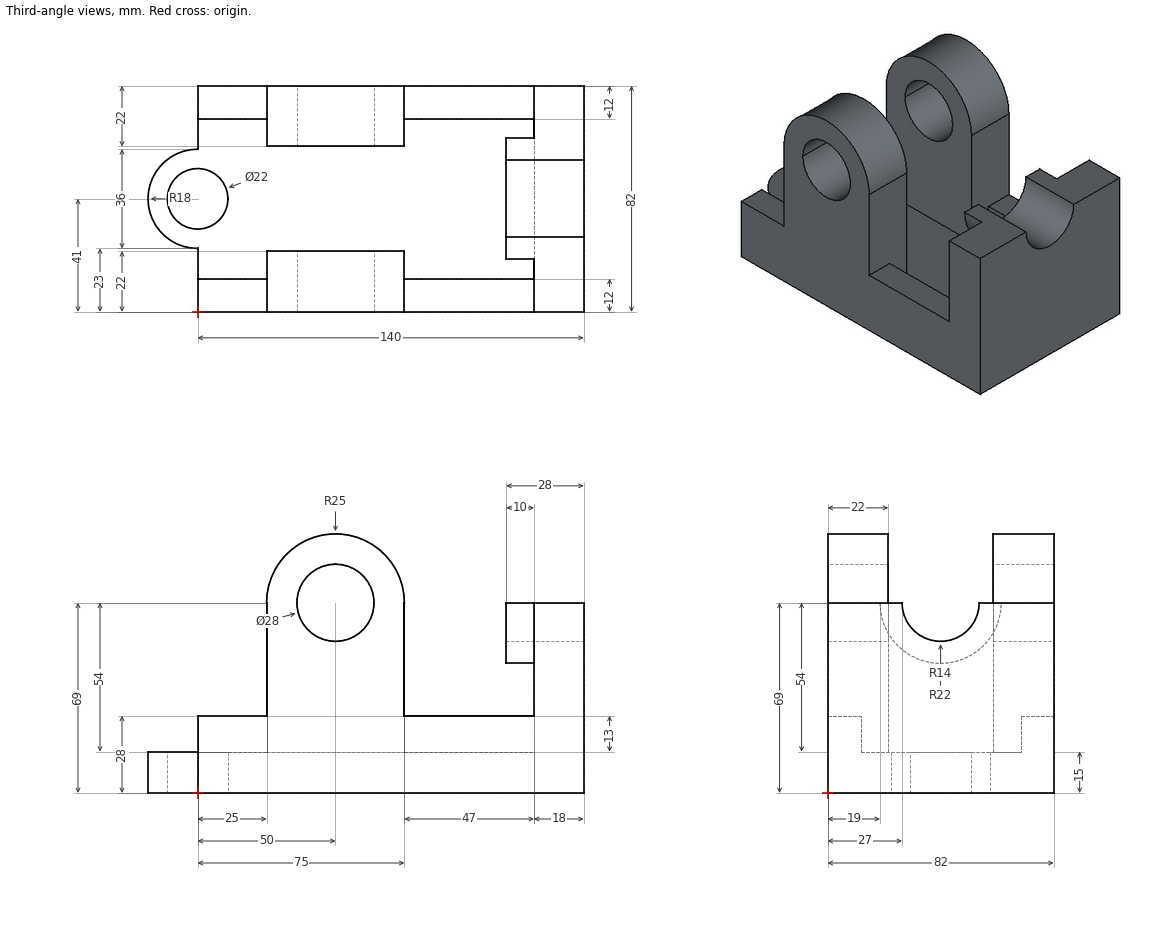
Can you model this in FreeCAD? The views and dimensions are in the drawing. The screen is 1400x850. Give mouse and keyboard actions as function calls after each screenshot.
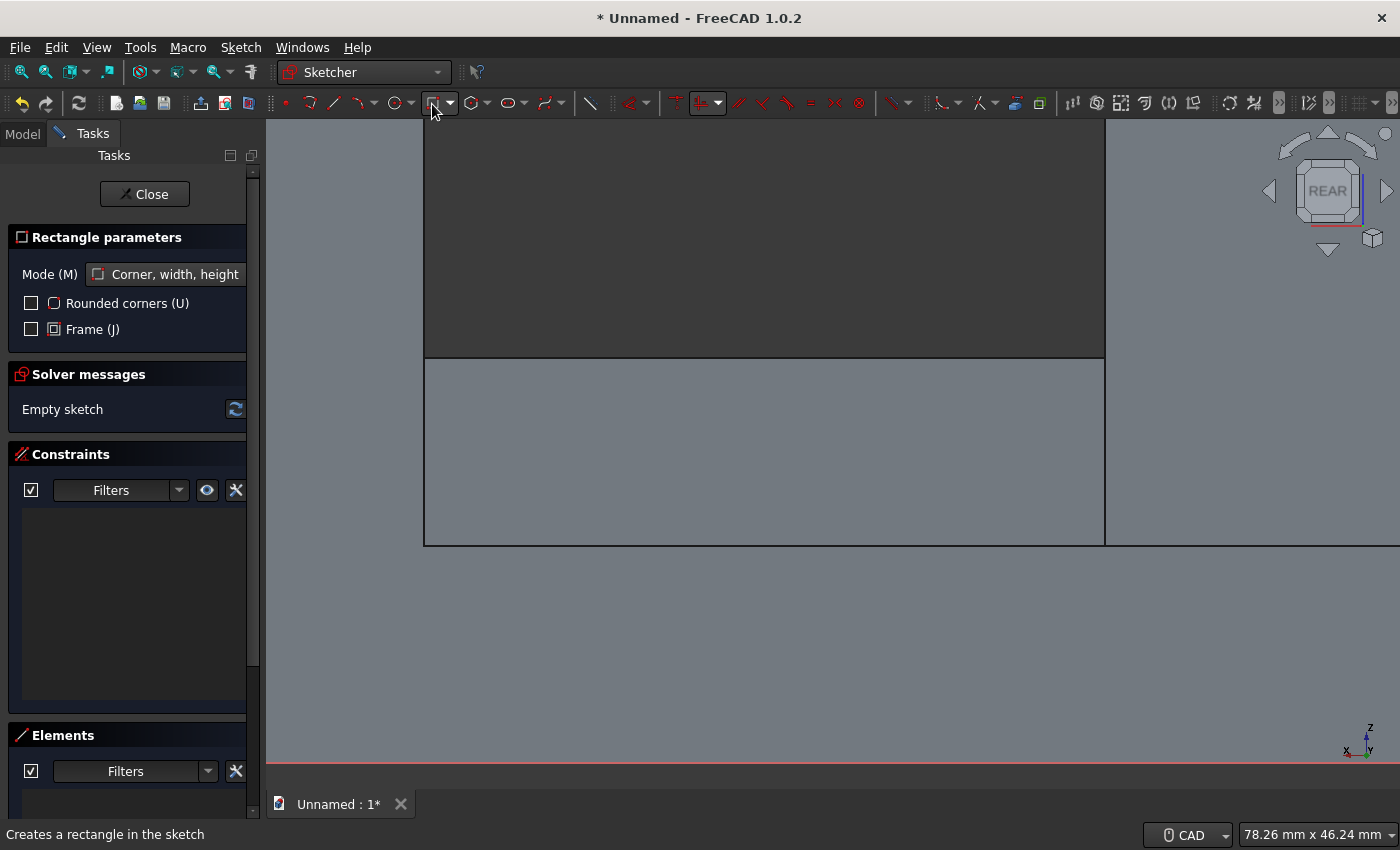
click(424, 358)
click(1105, 546)
key(Escape)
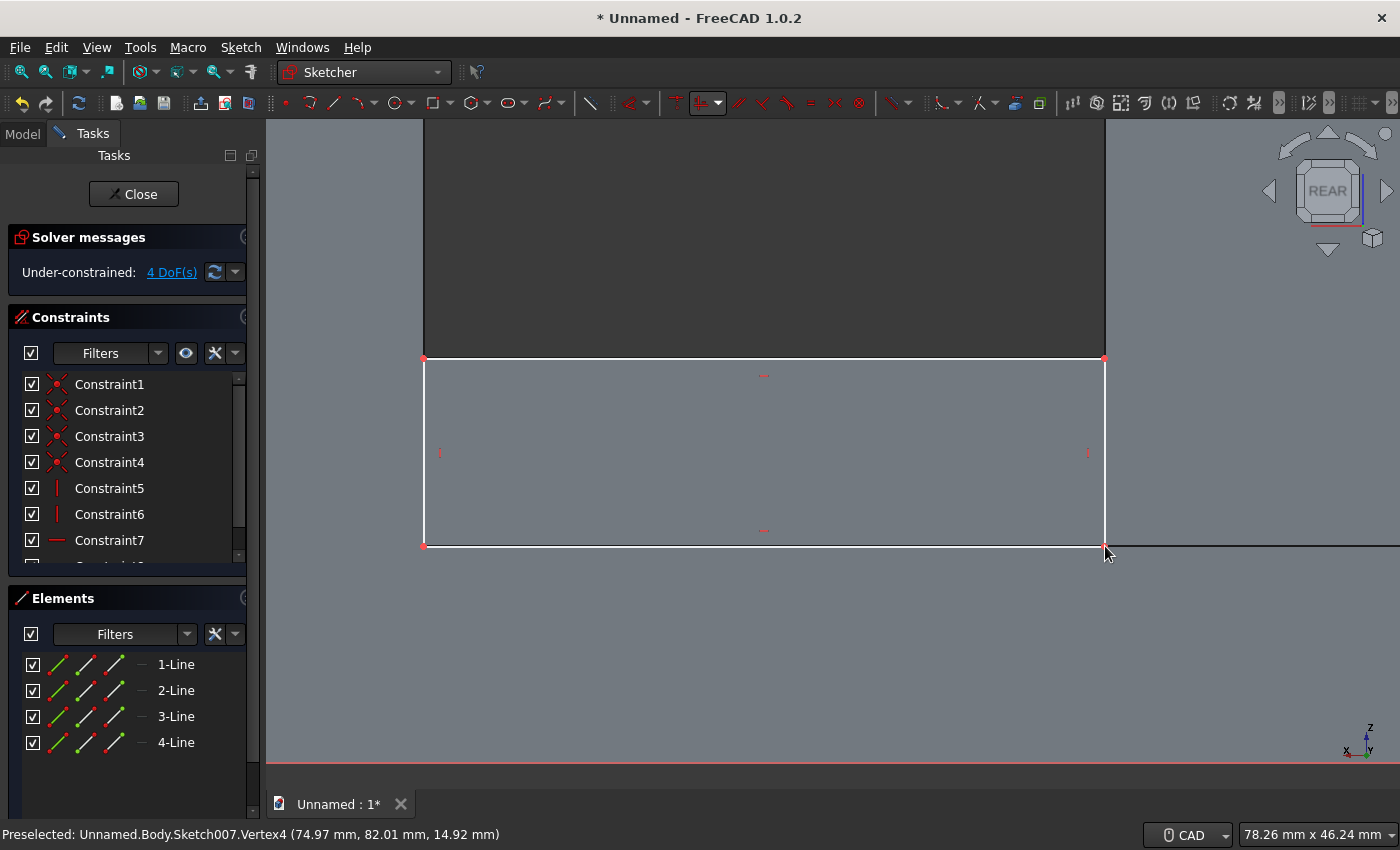
click(630, 104)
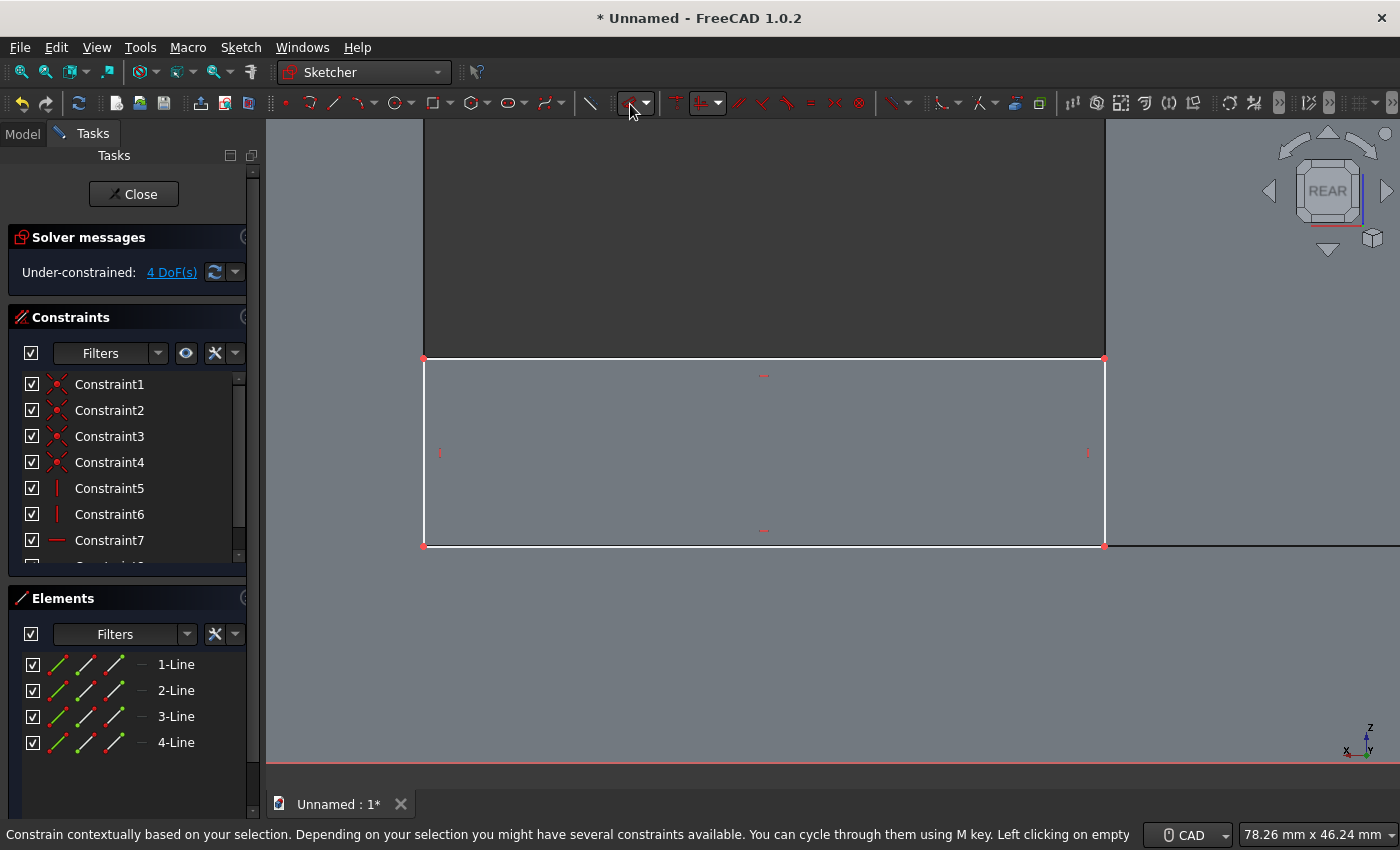
click(424, 415)
click(390, 453)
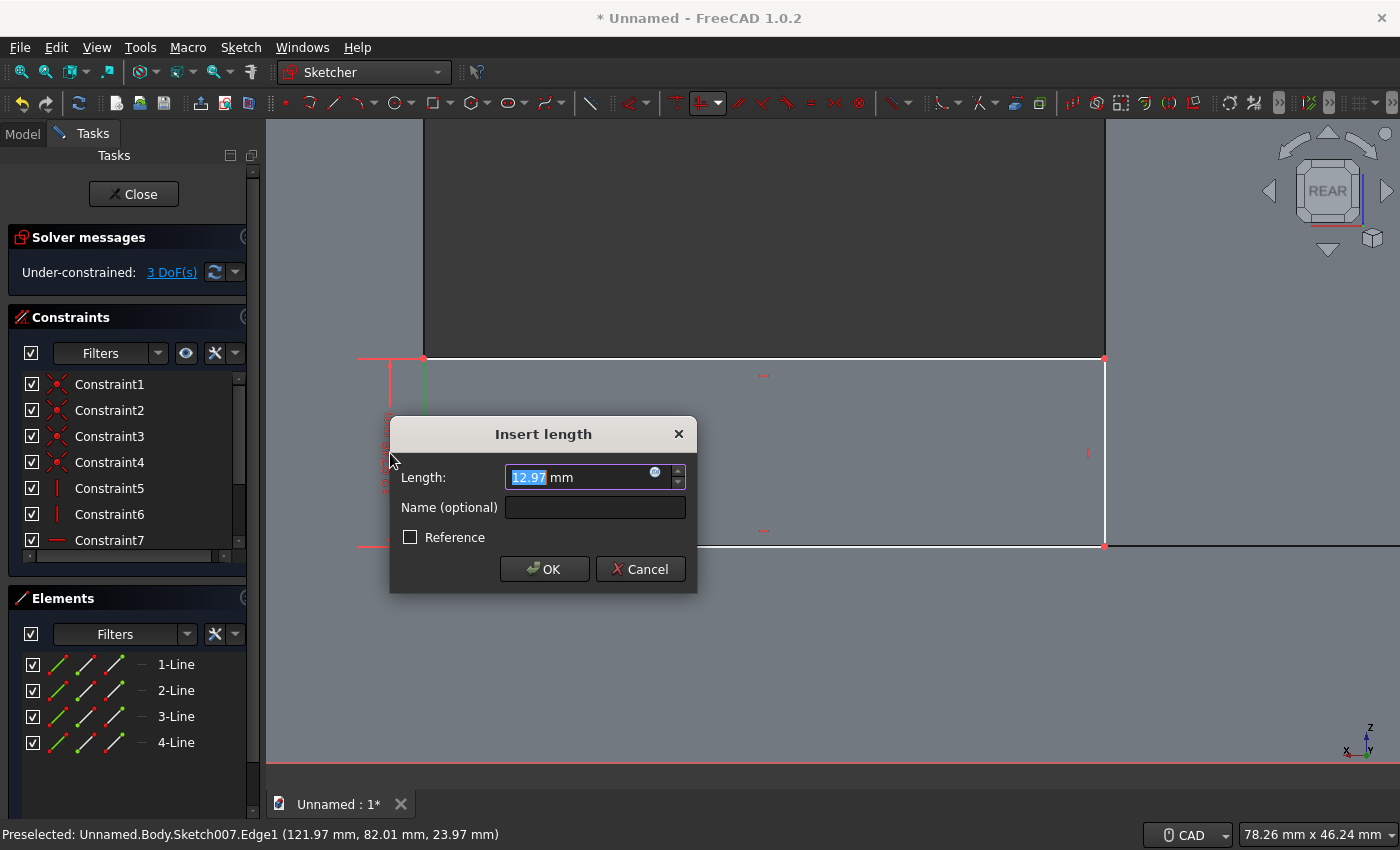
text(13)
key(Return)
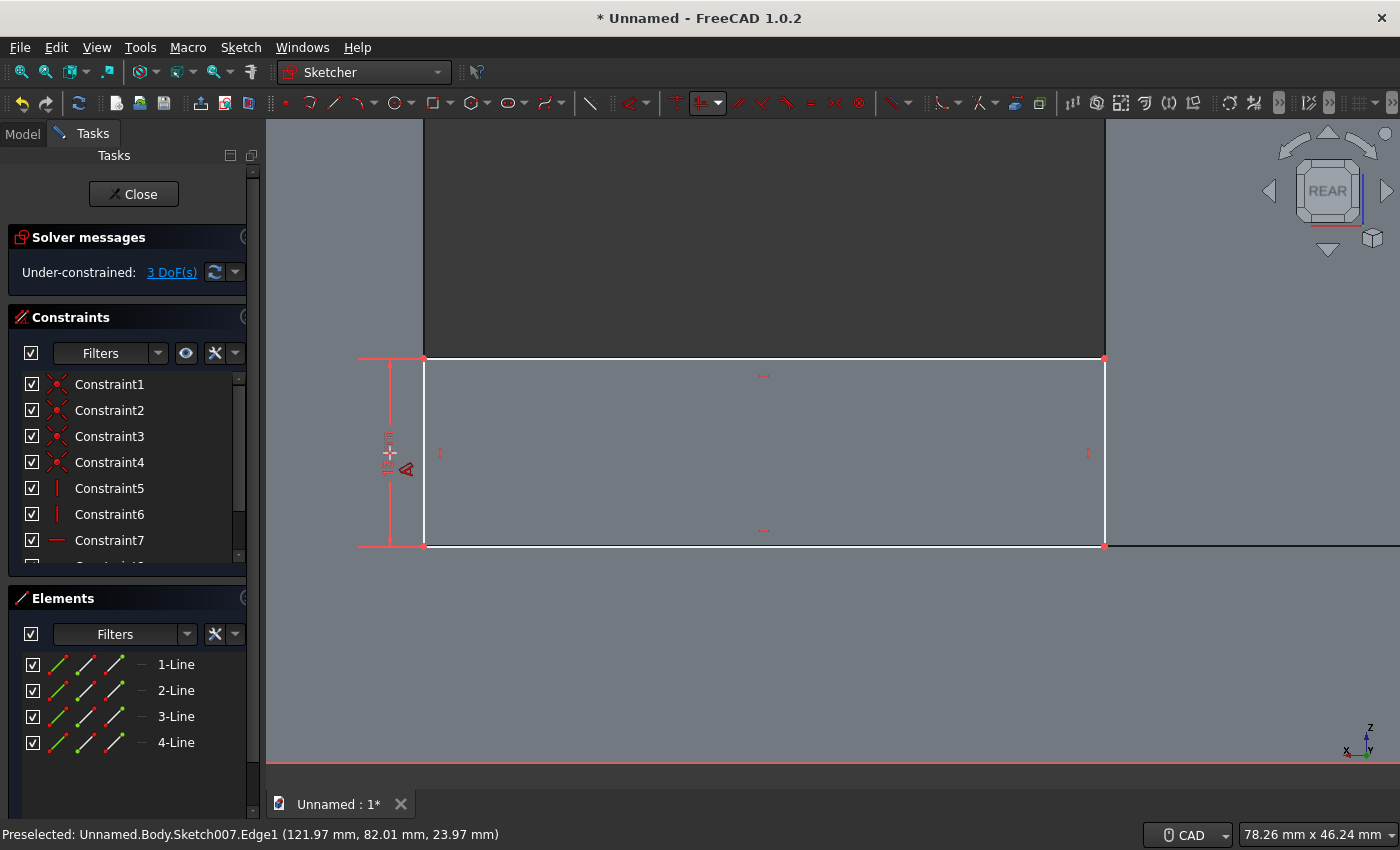
click(628, 547)
click(765, 581)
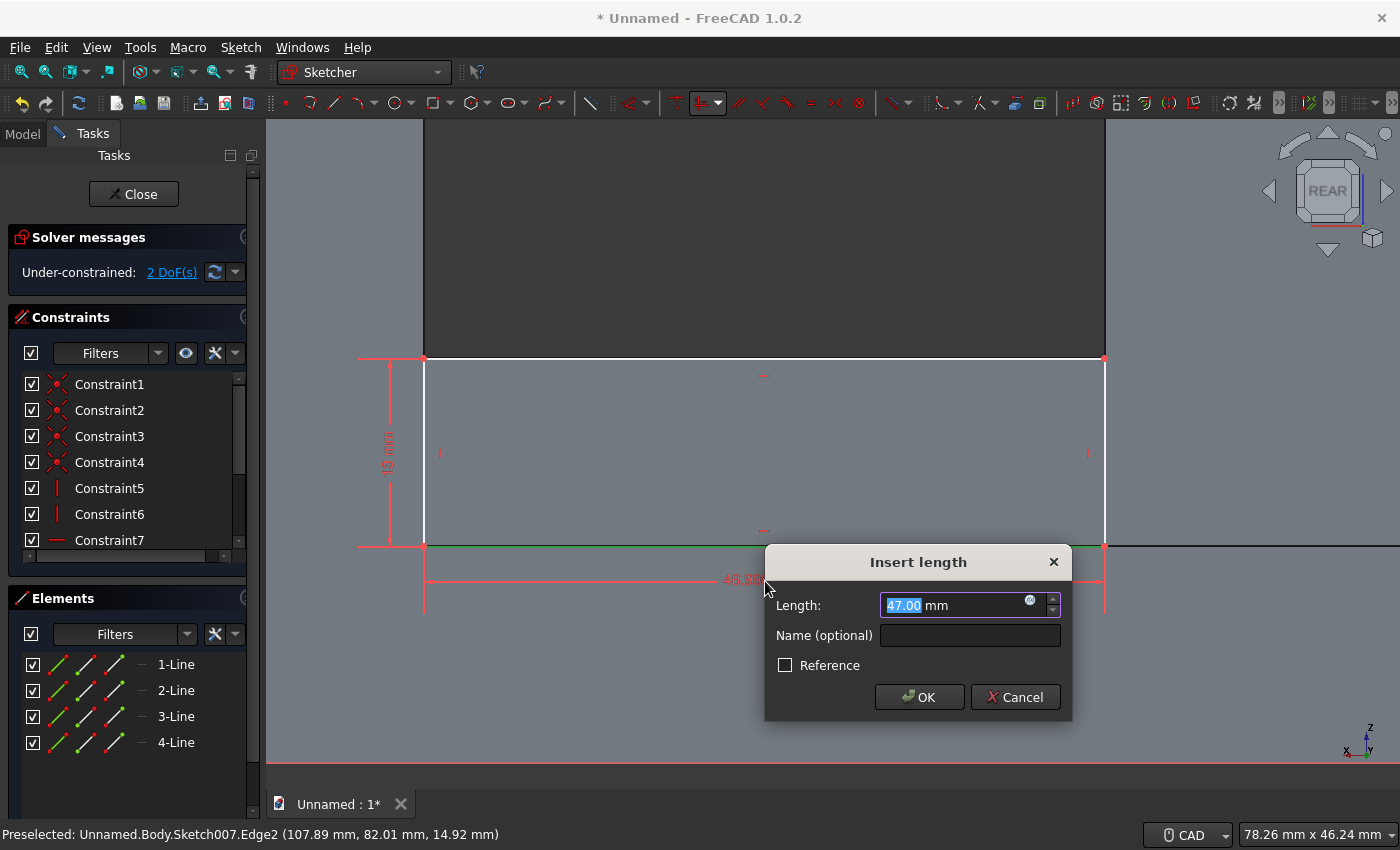
text(47)
key(Return)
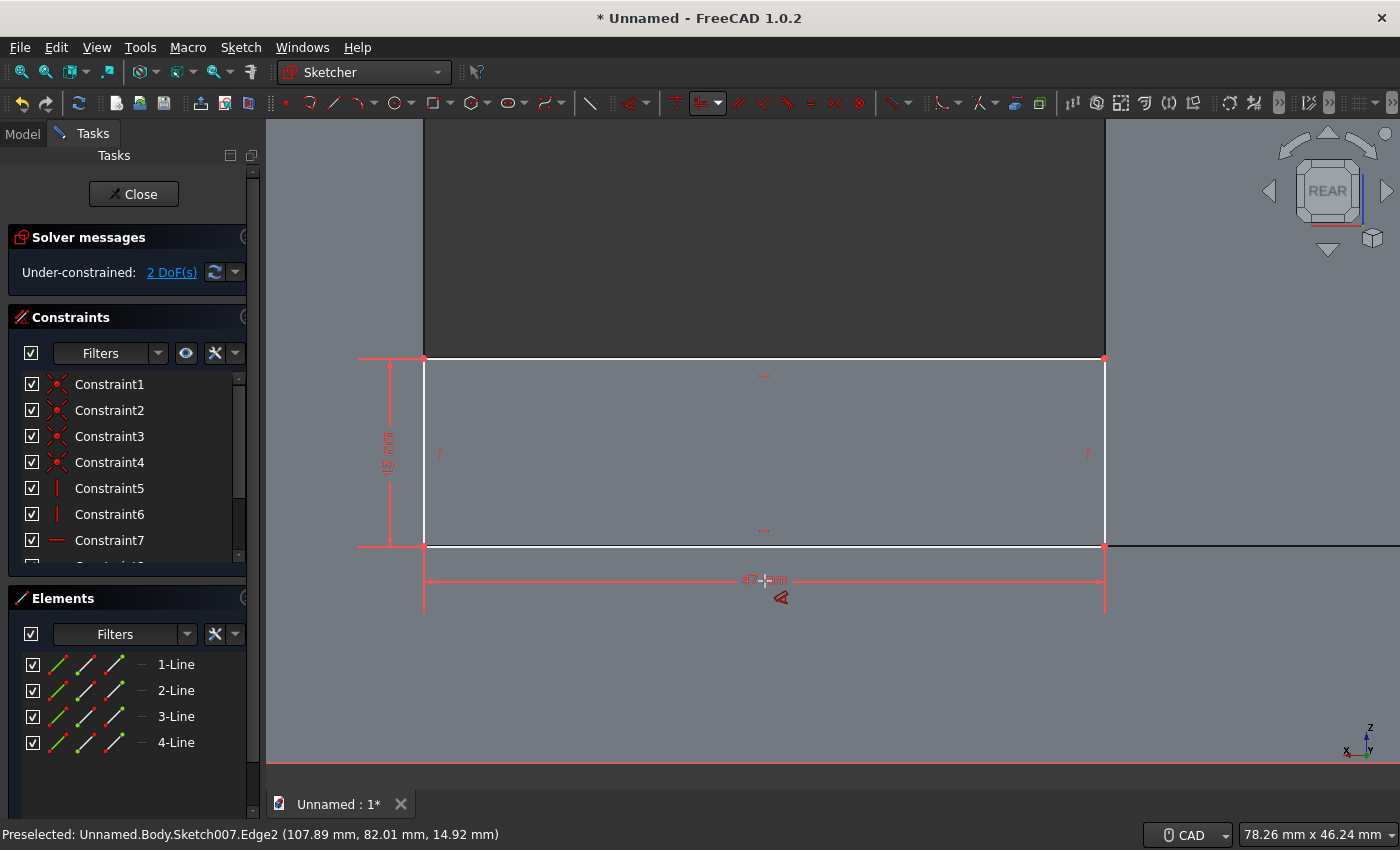
click(424, 359)
click(390, 560)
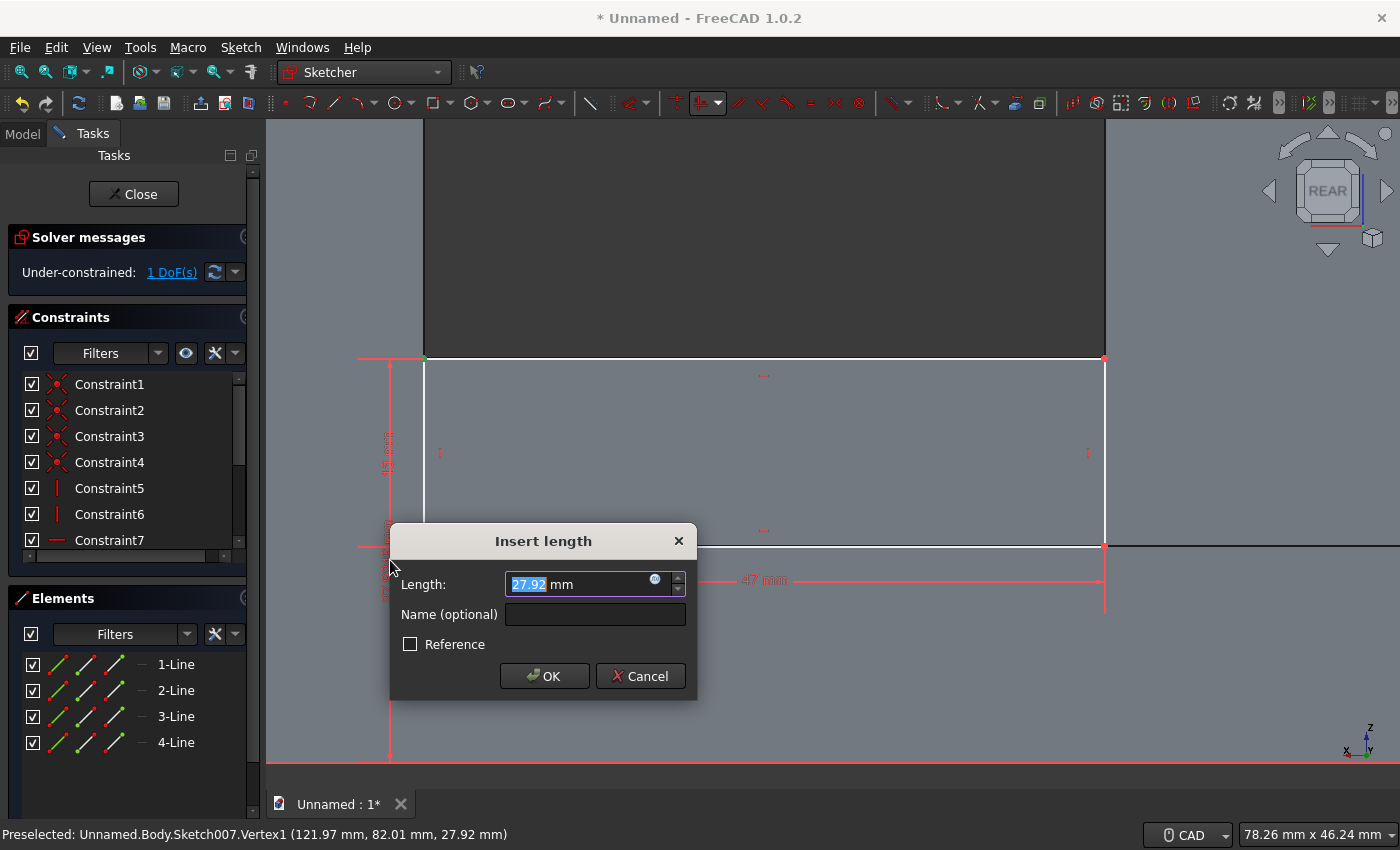
text(28)
key(Return)